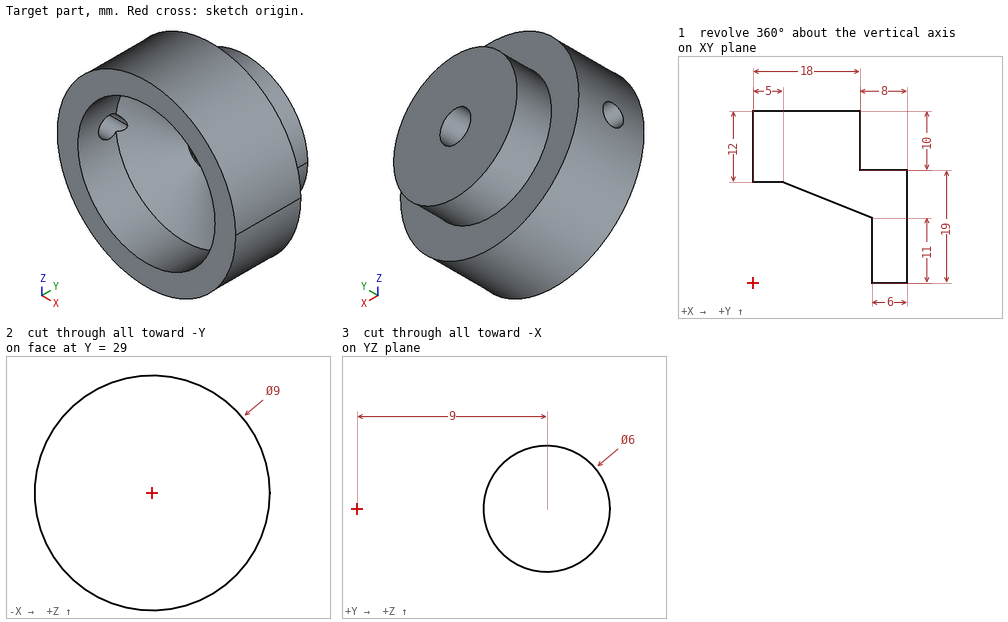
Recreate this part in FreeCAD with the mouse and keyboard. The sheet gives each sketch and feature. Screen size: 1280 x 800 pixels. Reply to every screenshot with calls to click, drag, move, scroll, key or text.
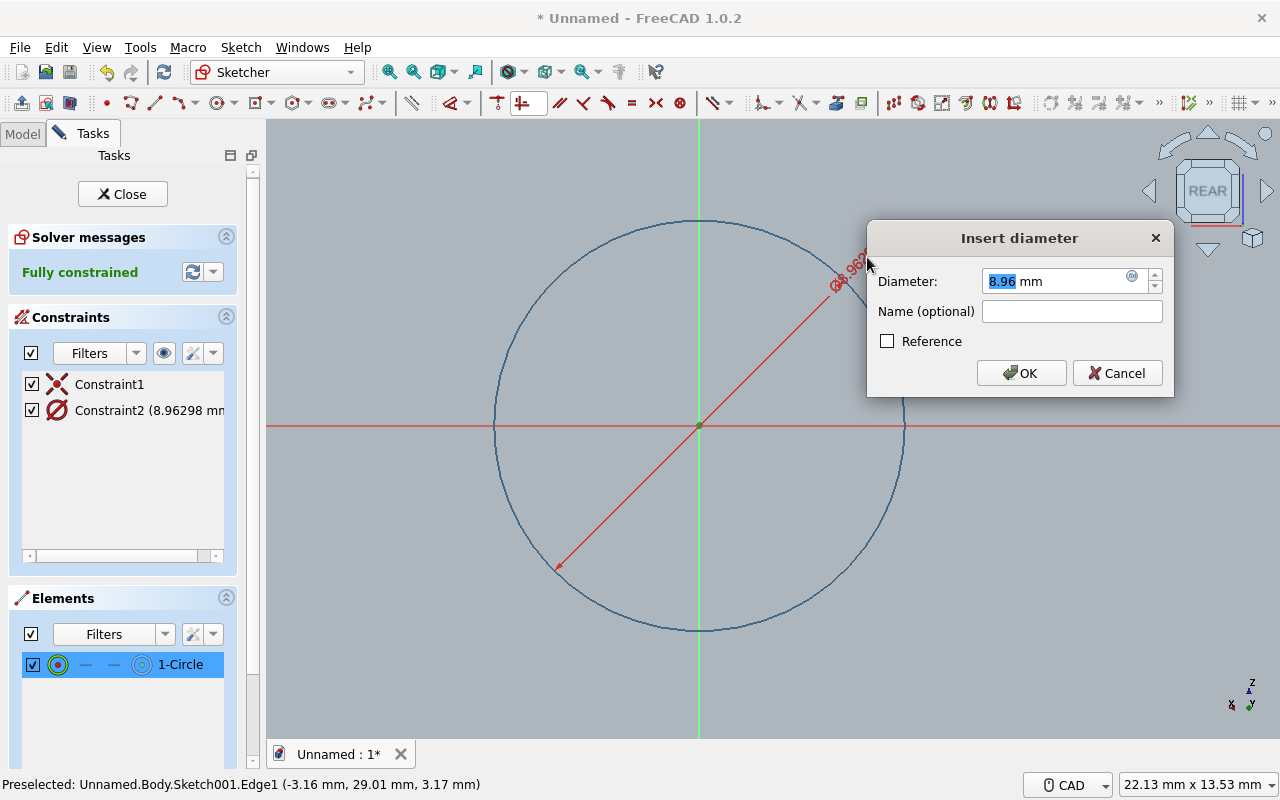
text(9)
key(Return)
key(Escape)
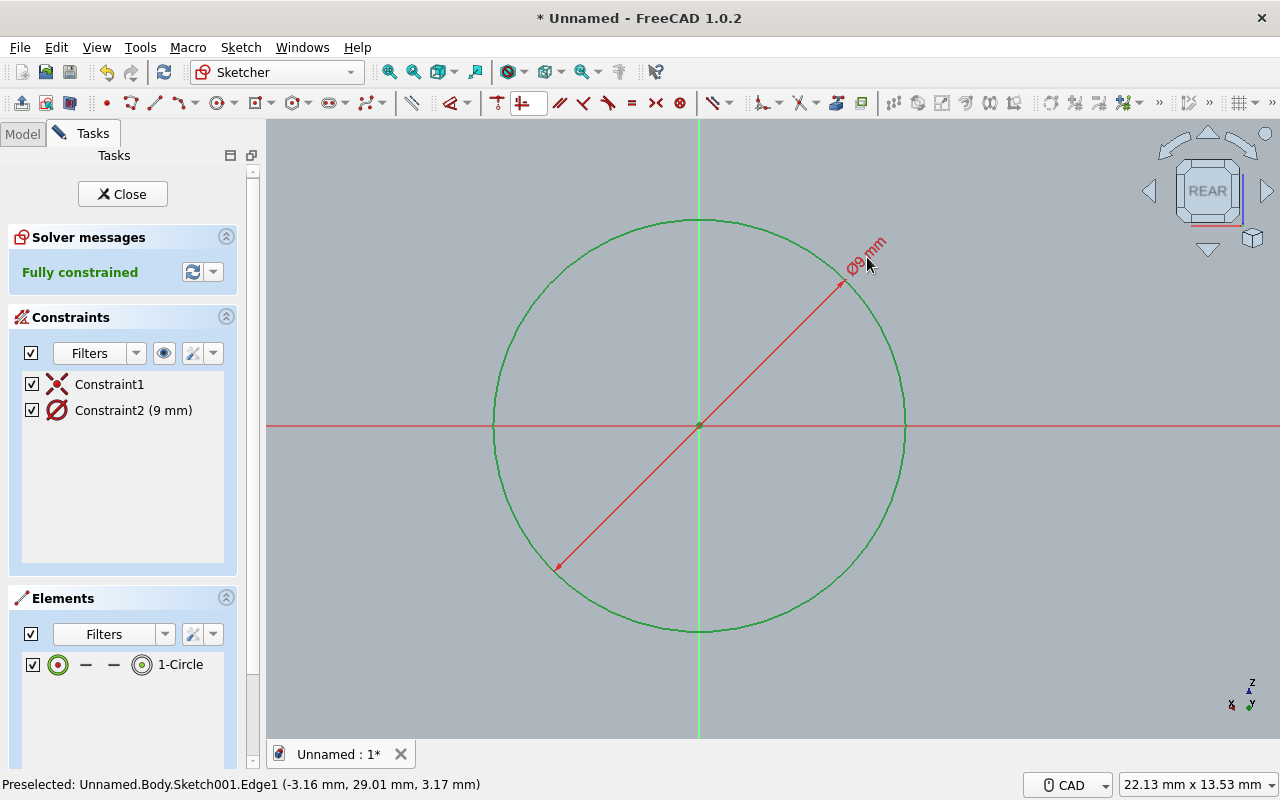
click(123, 194)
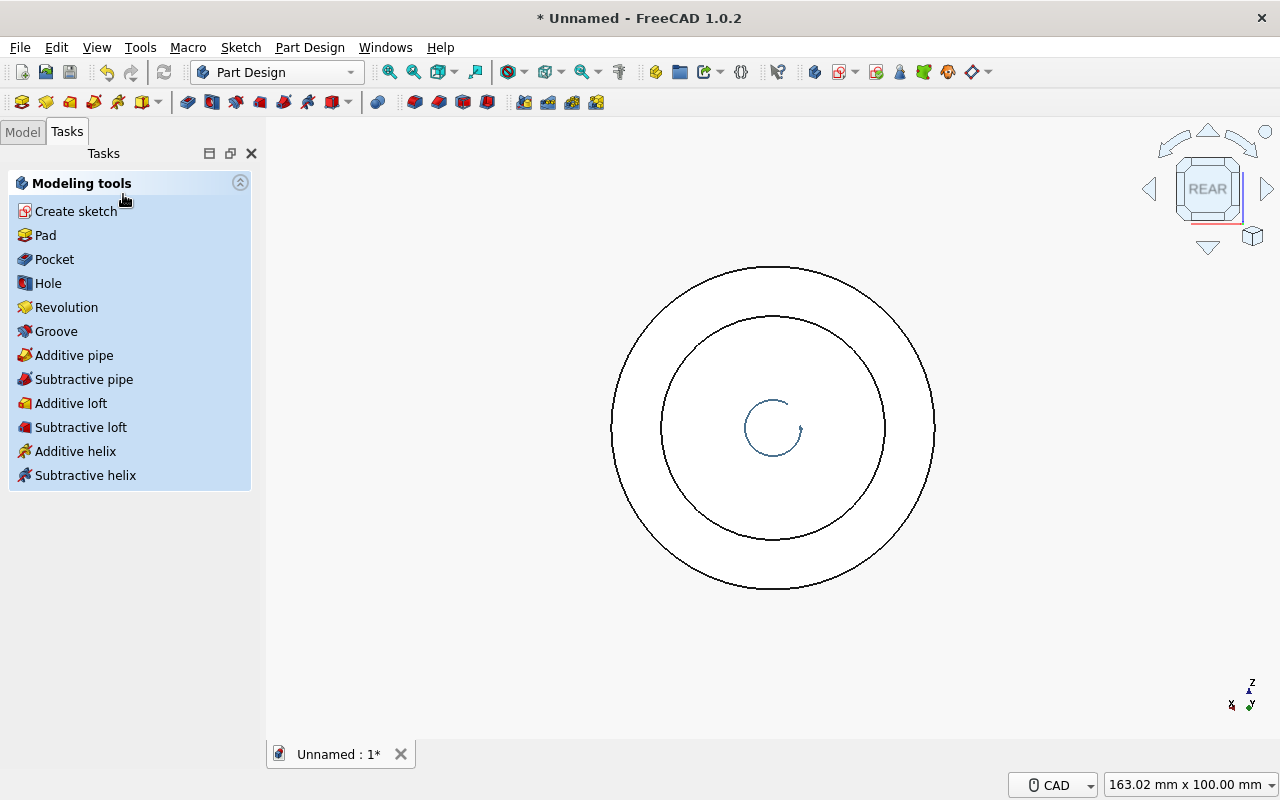
click(188, 102)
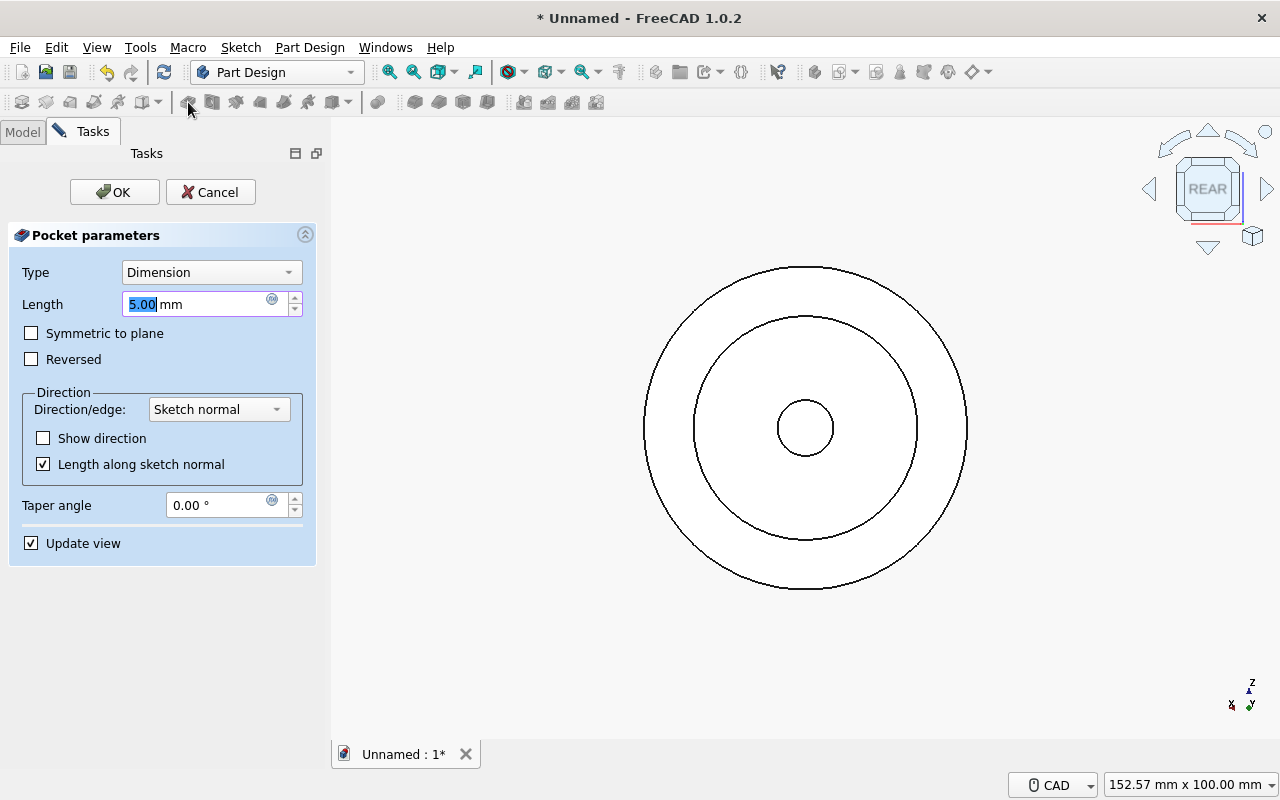
click(212, 272)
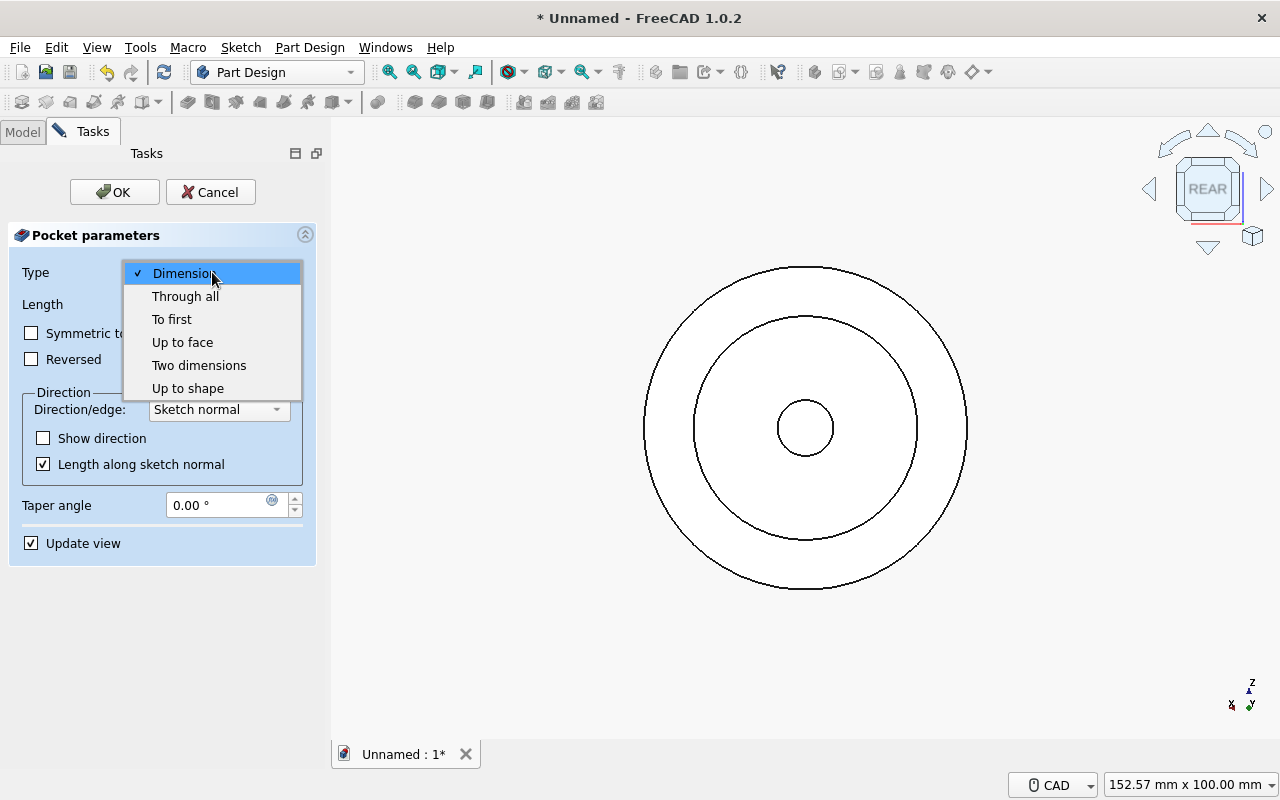
click(212, 296)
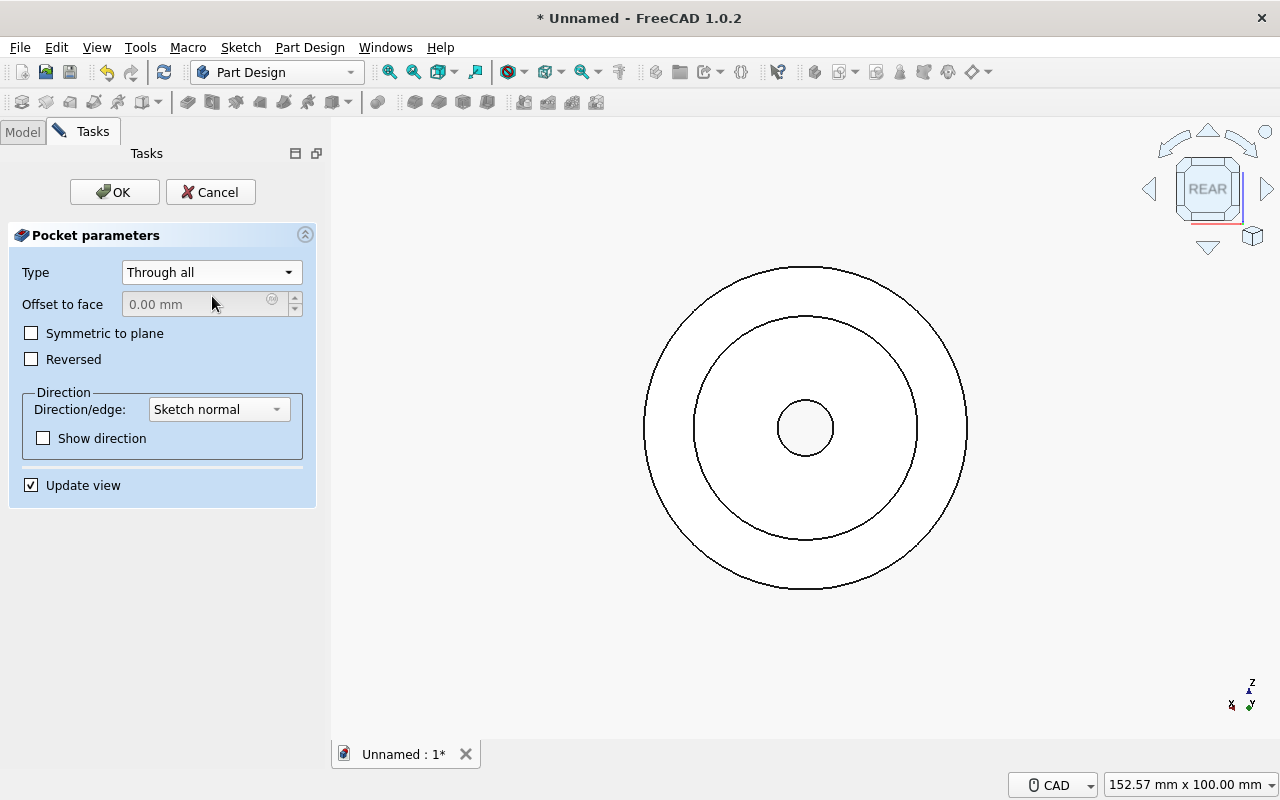
click(115, 192)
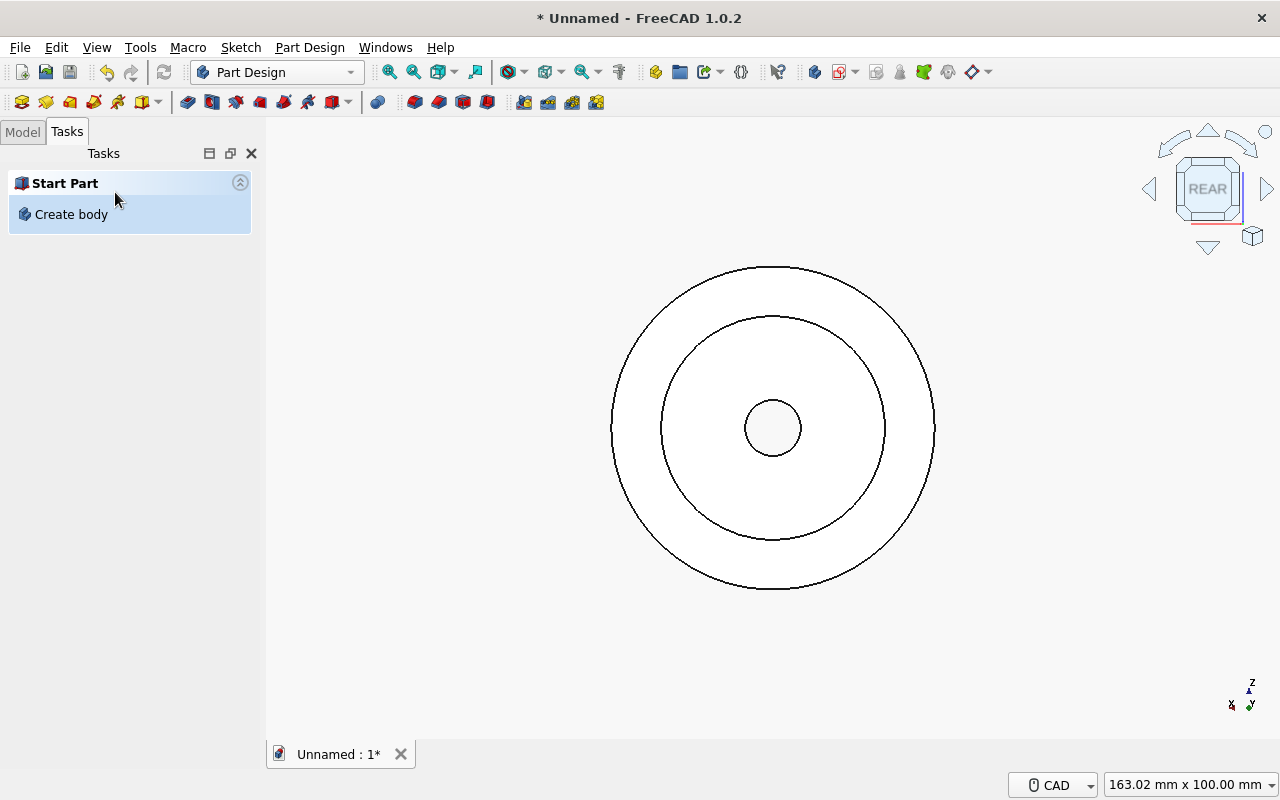
click(840, 72)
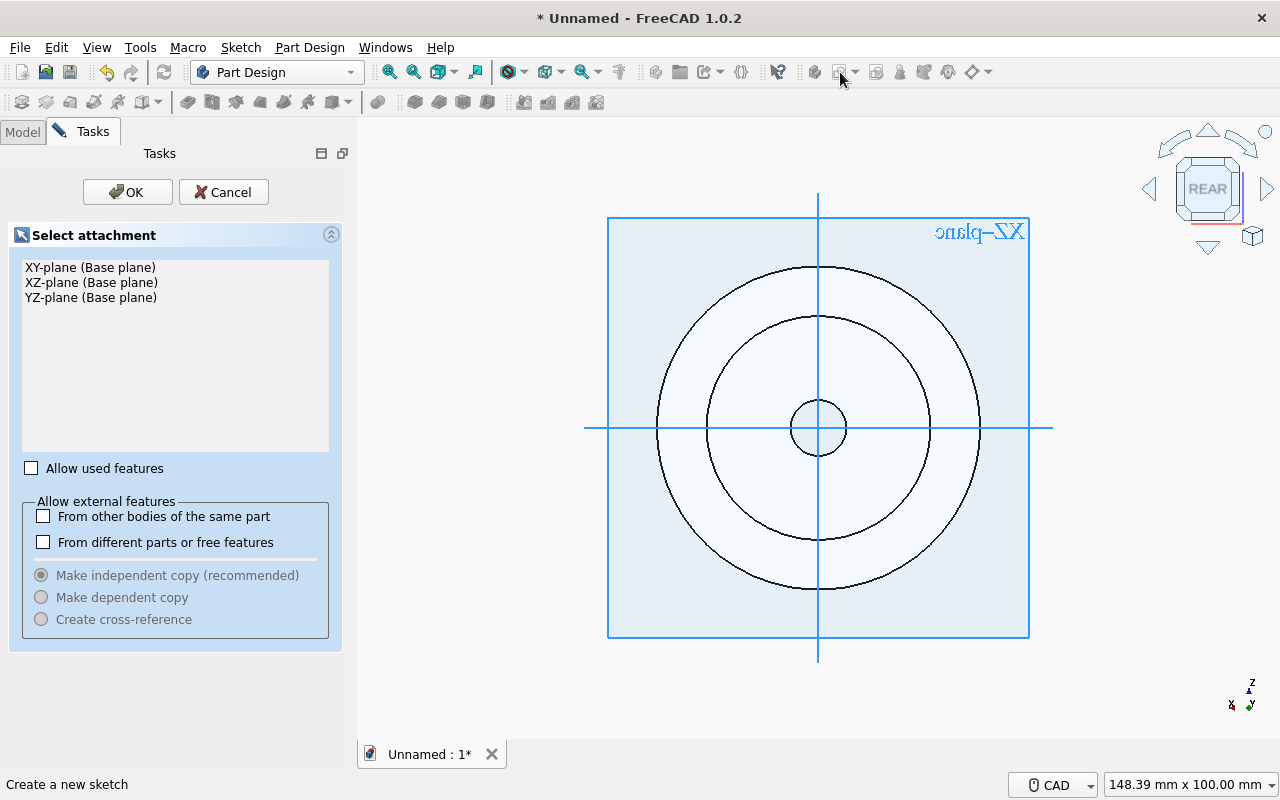
click(82, 298)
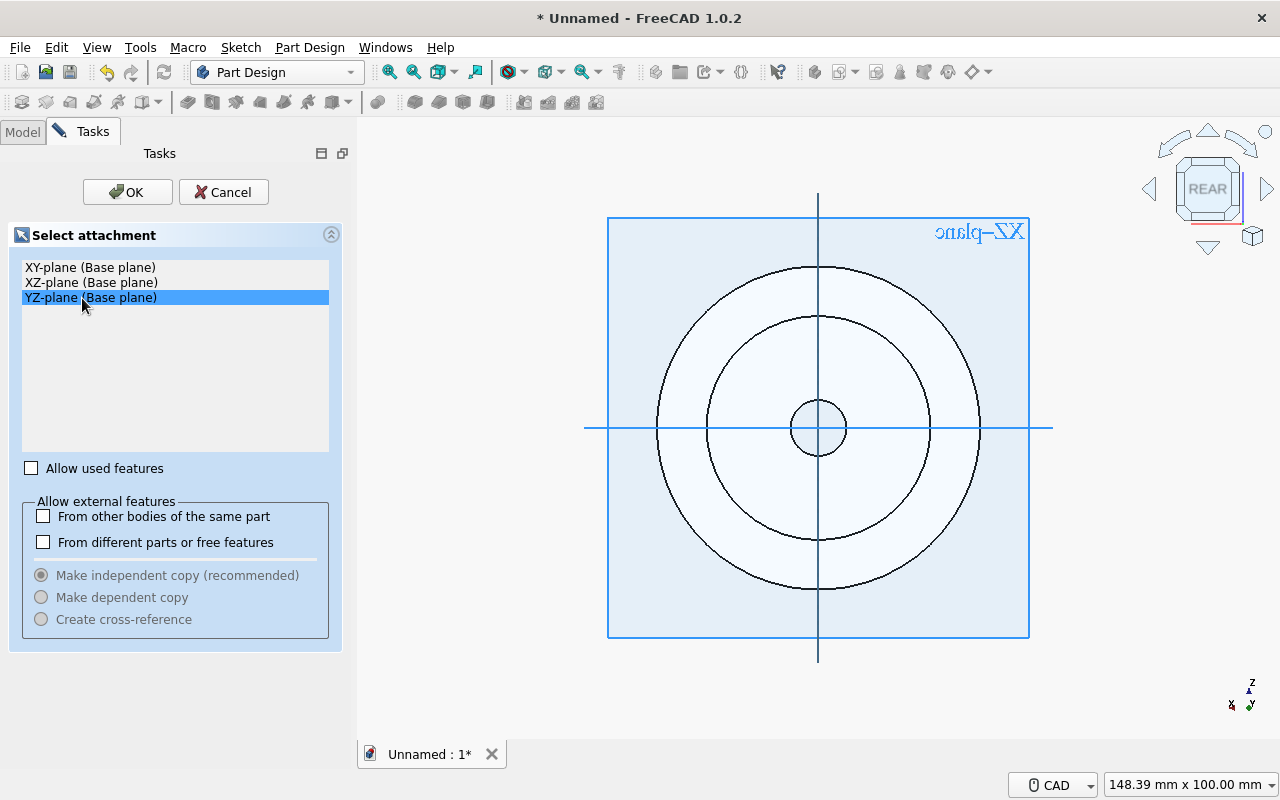
click(128, 192)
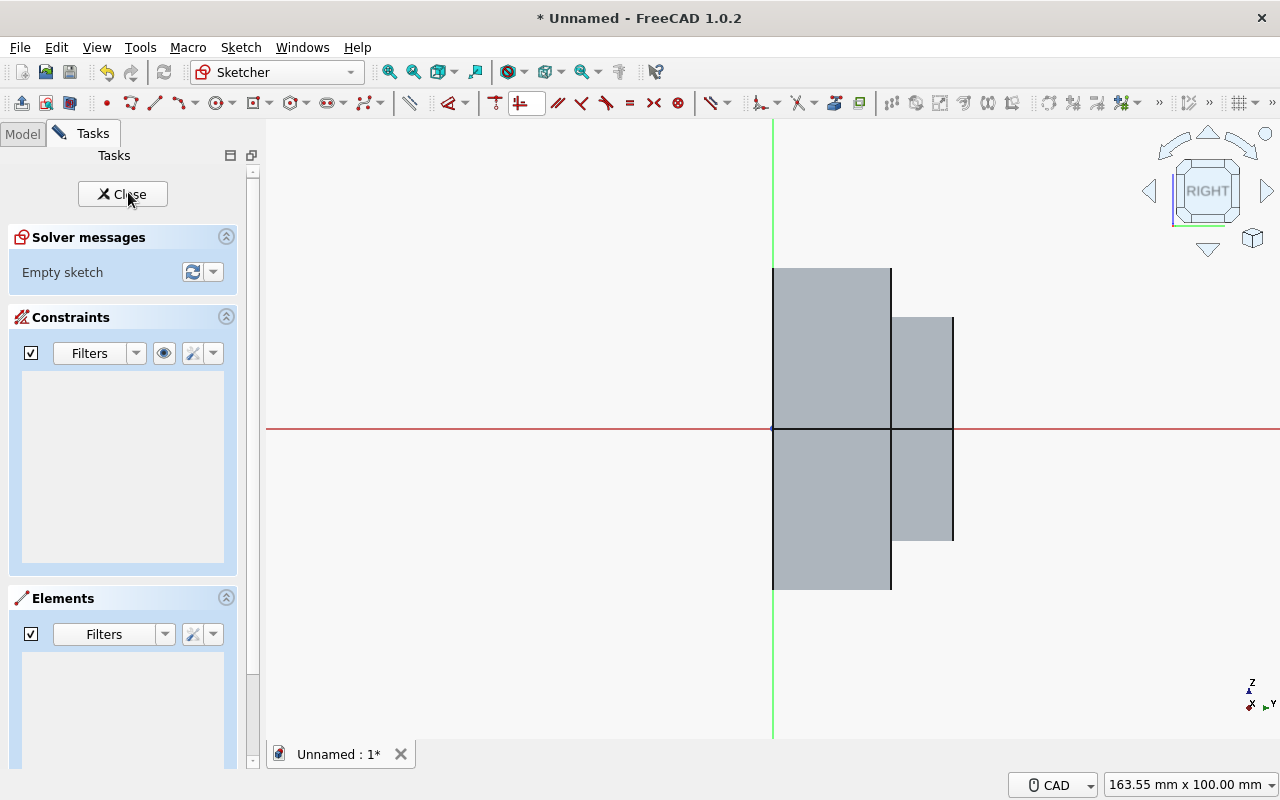
click(70, 104)